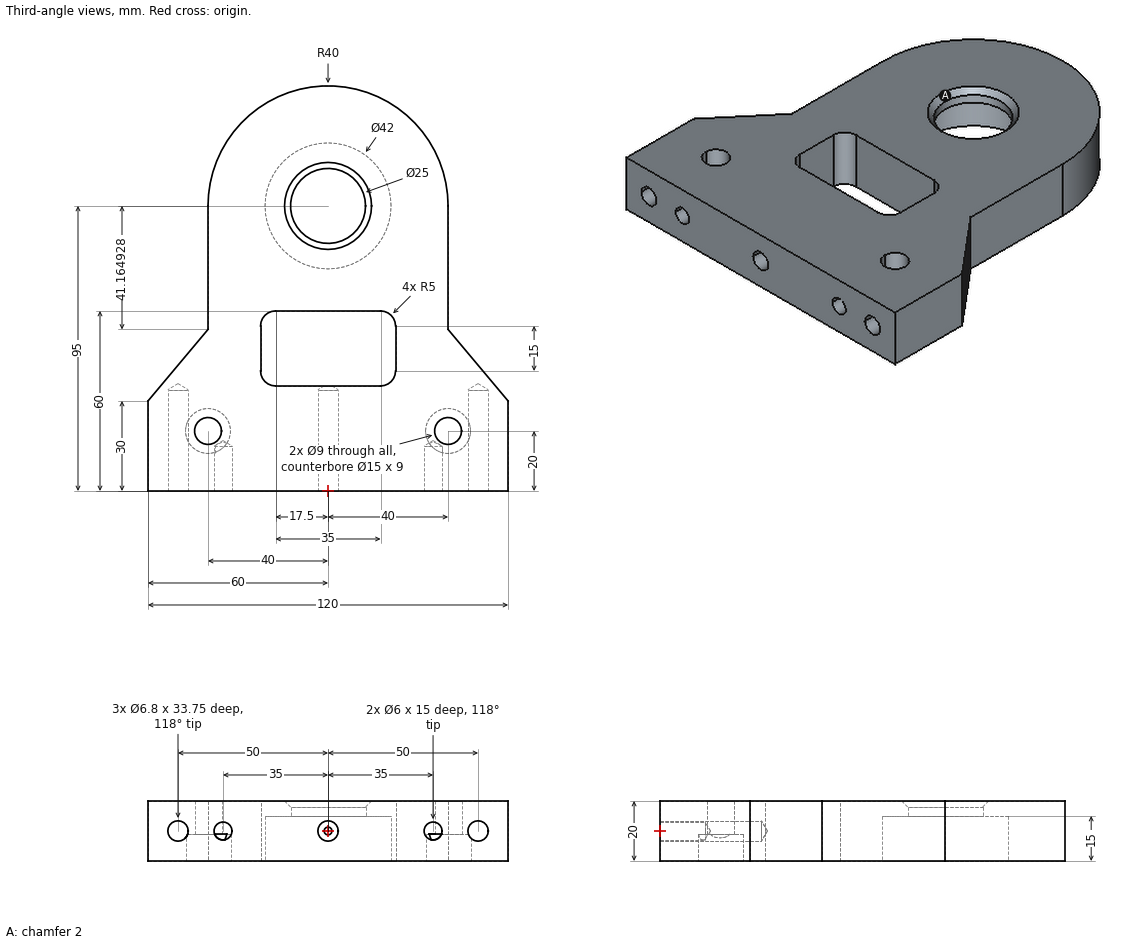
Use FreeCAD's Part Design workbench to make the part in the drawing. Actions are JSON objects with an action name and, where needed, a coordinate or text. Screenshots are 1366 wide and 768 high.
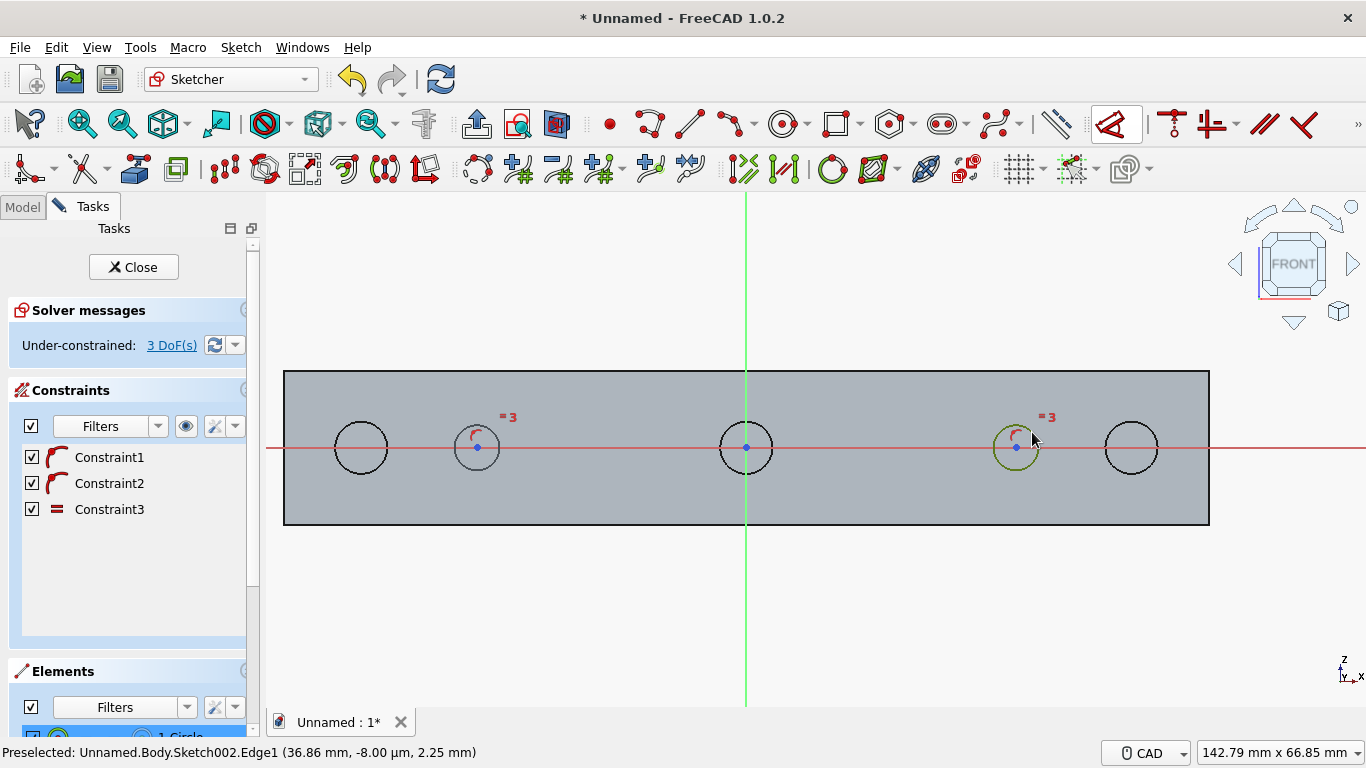
{"action": "left_click", "coordinate": [1136, 124]}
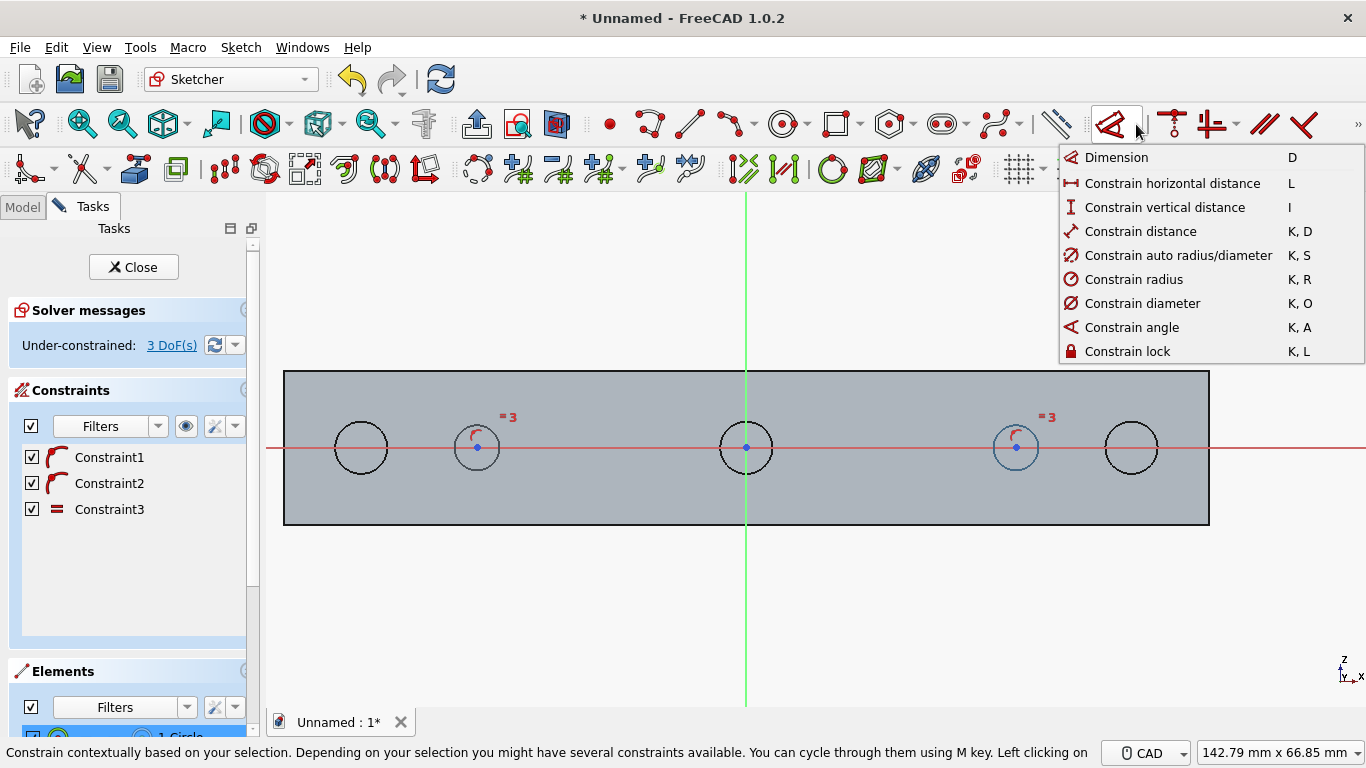
{"action": "left_click", "coordinate": [1212, 303]}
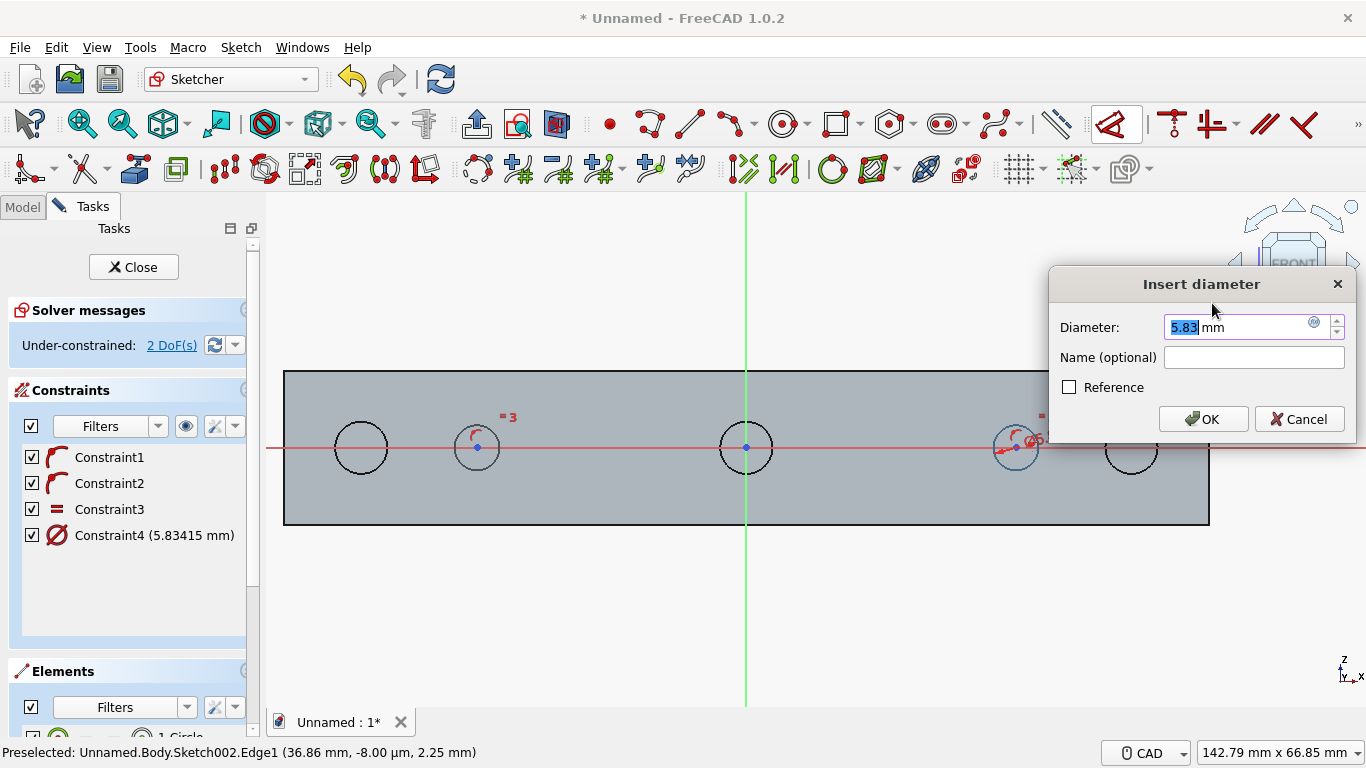
{"action": "type", "text": "6"}
{"action": "key", "text": "Return"}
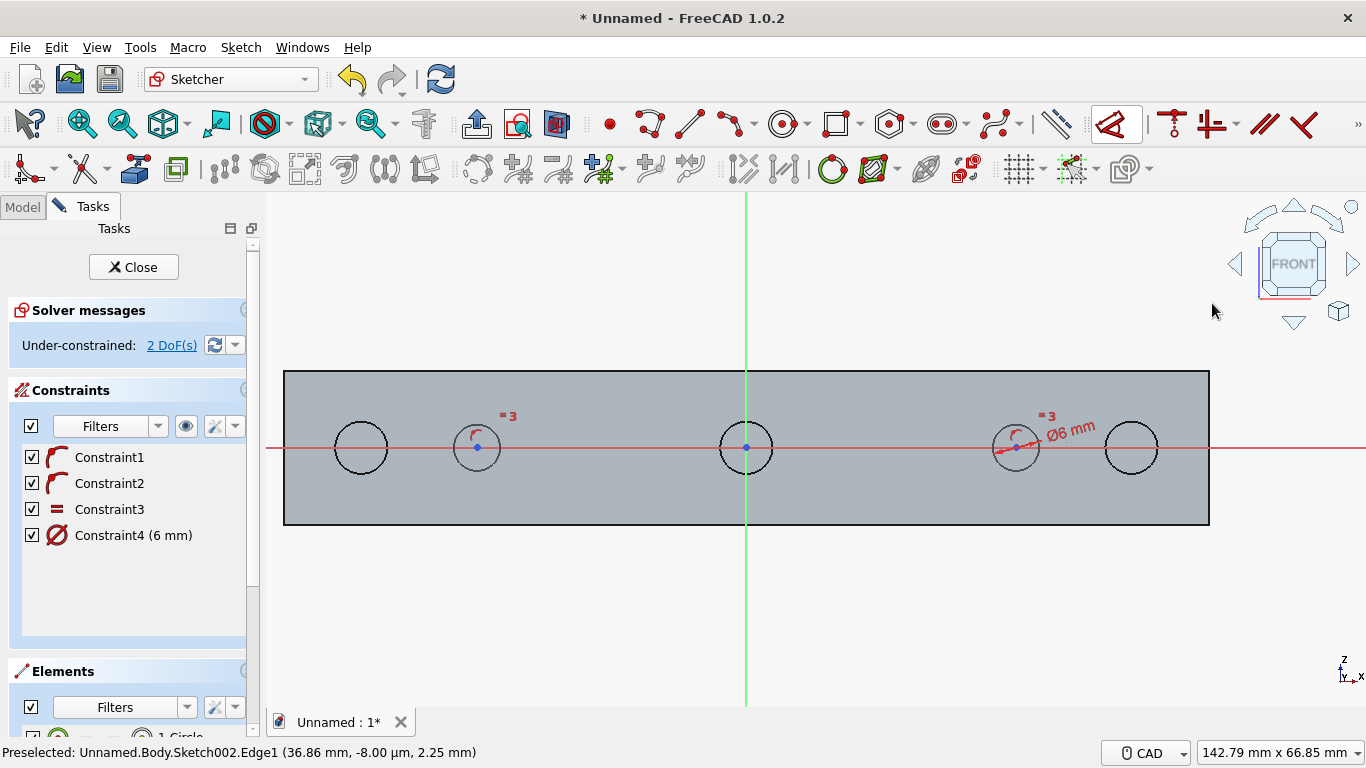
{"action": "left_click", "coordinate": [1016, 448]}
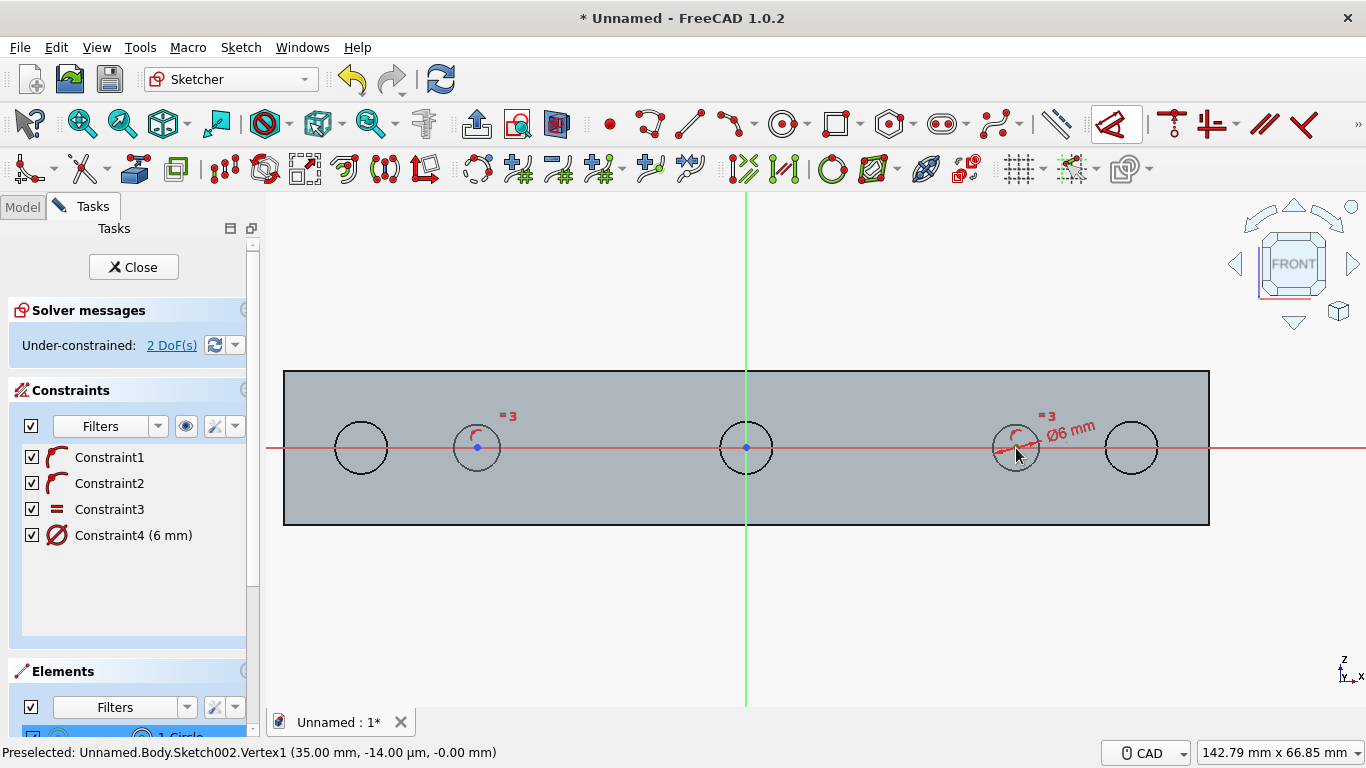
{"action": "left_click", "coordinate": [1136, 124]}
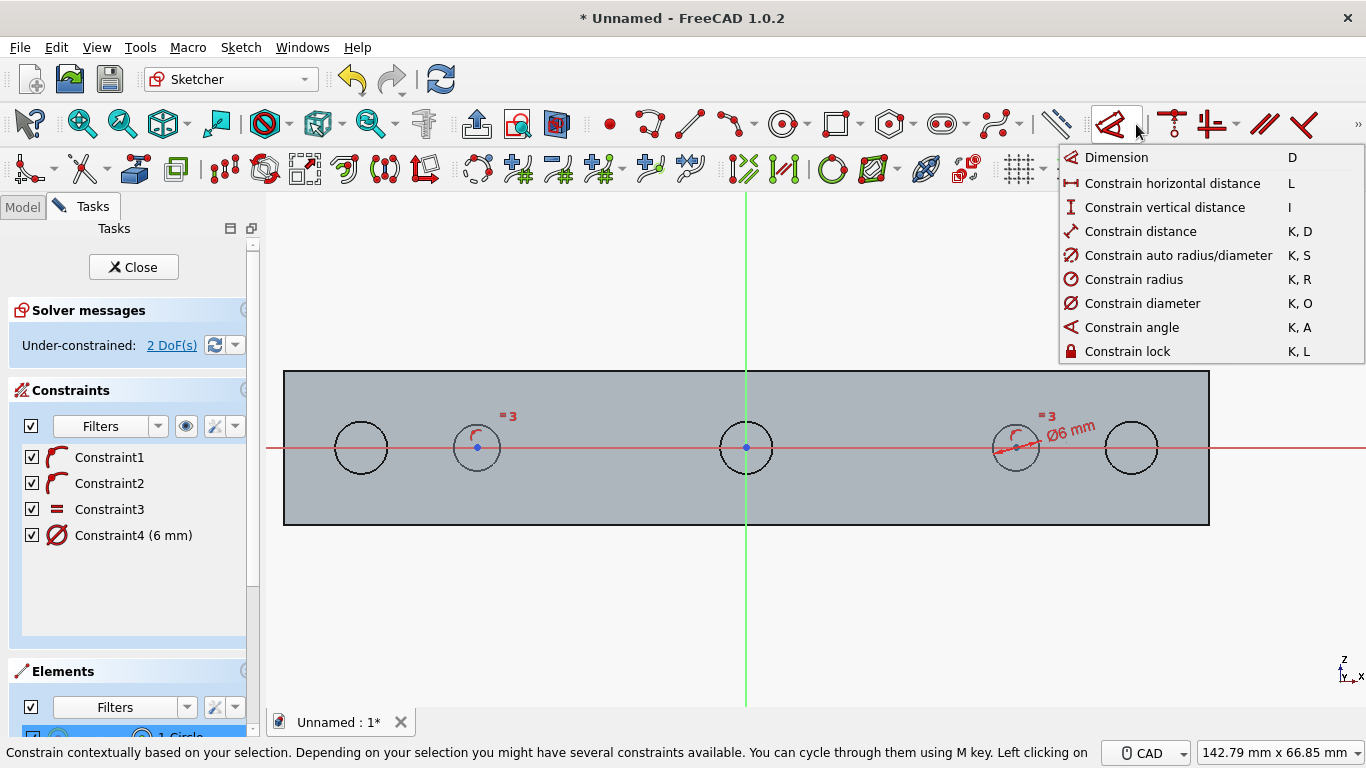
{"action": "left_click", "coordinate": [1212, 183]}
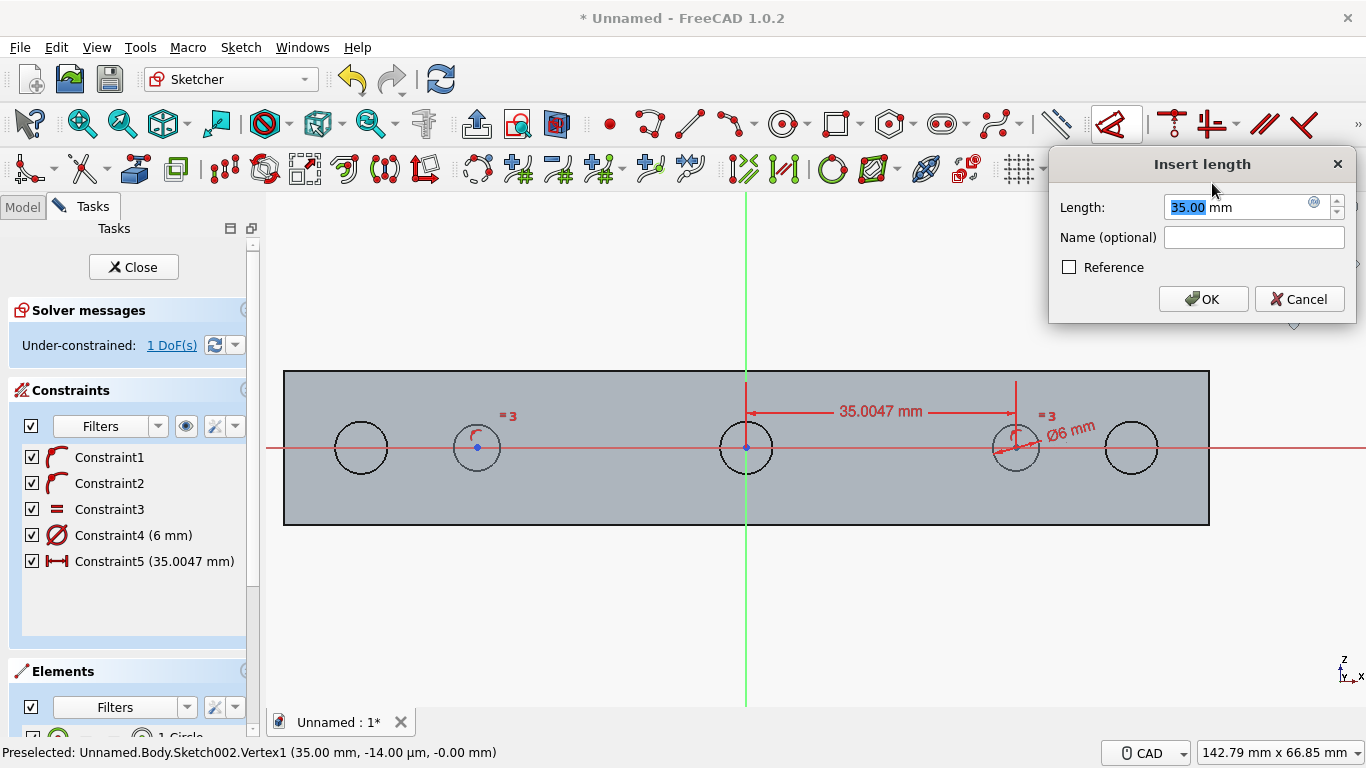
{"action": "type", "text": "35"}
{"action": "key", "text": "Return"}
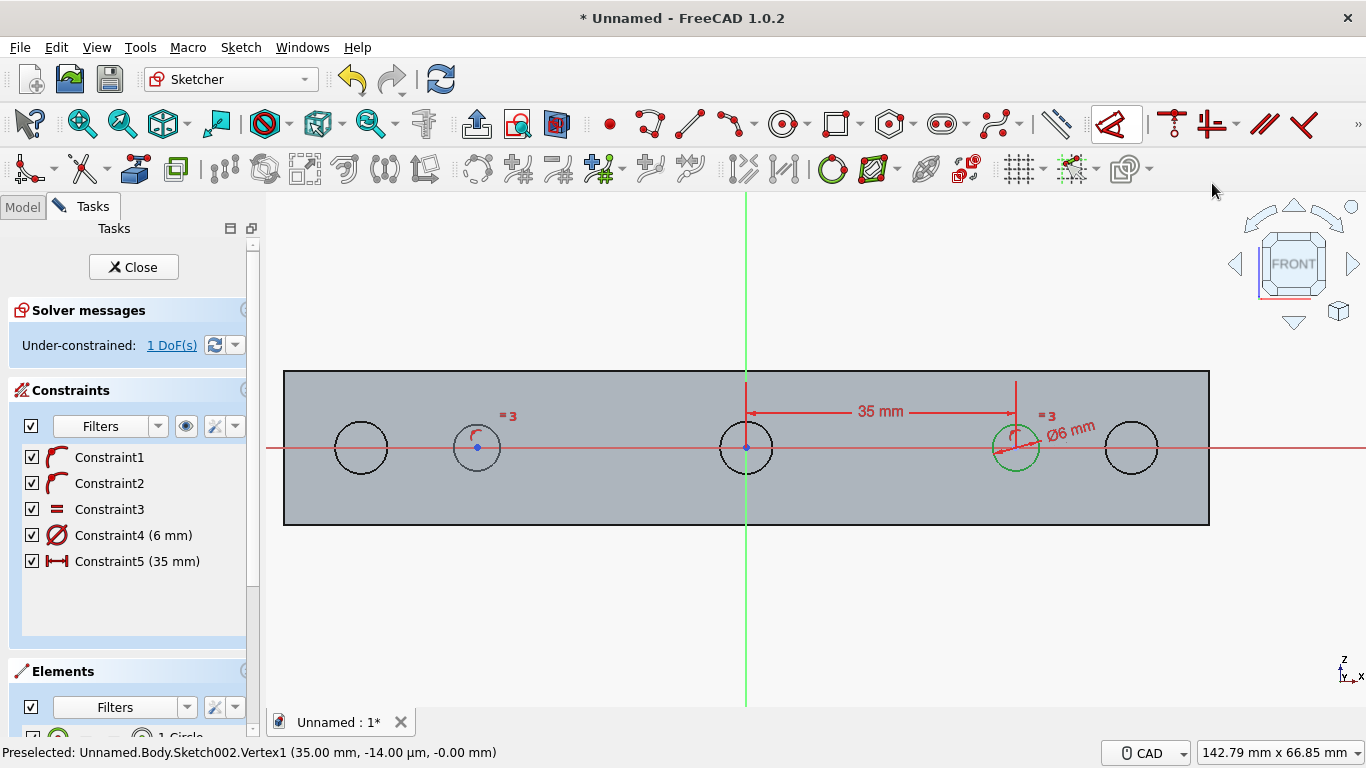
{"action": "left_click", "coordinate": [477, 448]}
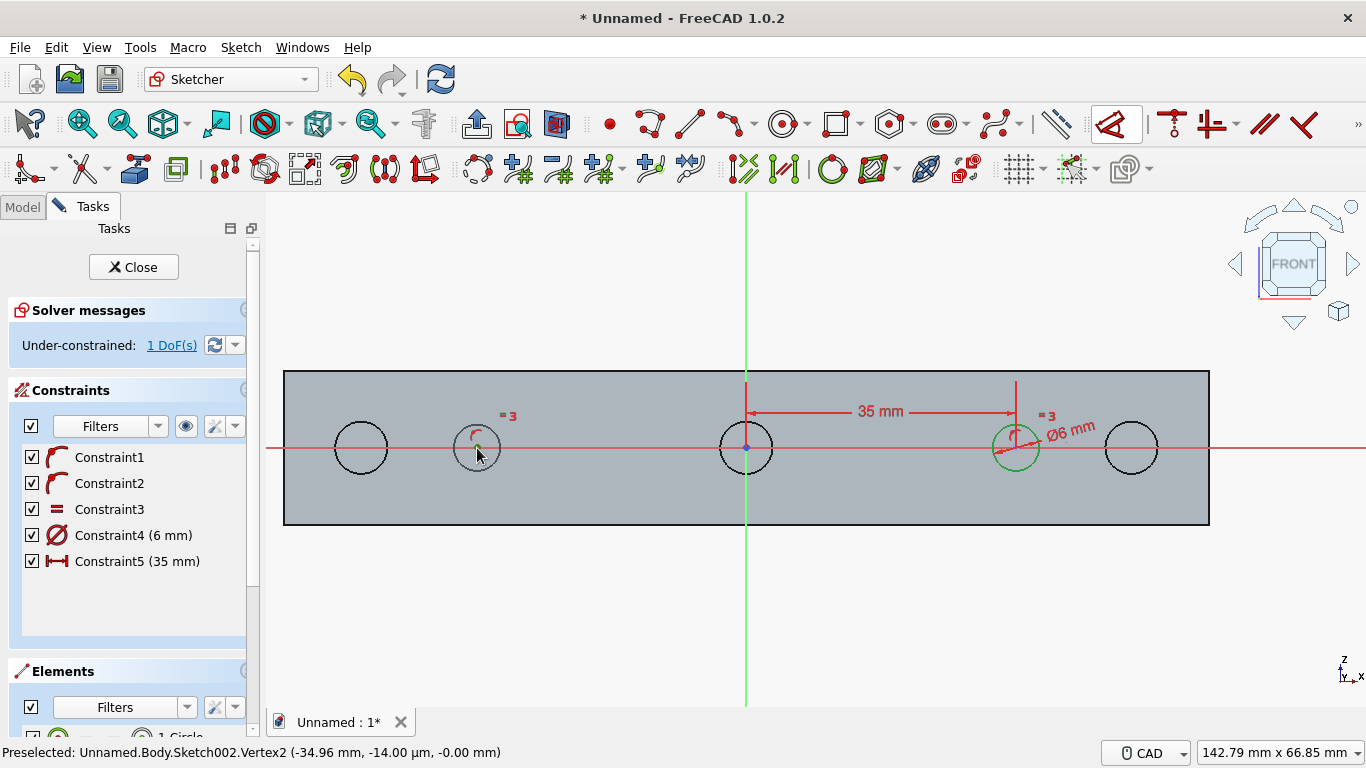
{"action": "left_click", "coordinate": [1136, 124]}